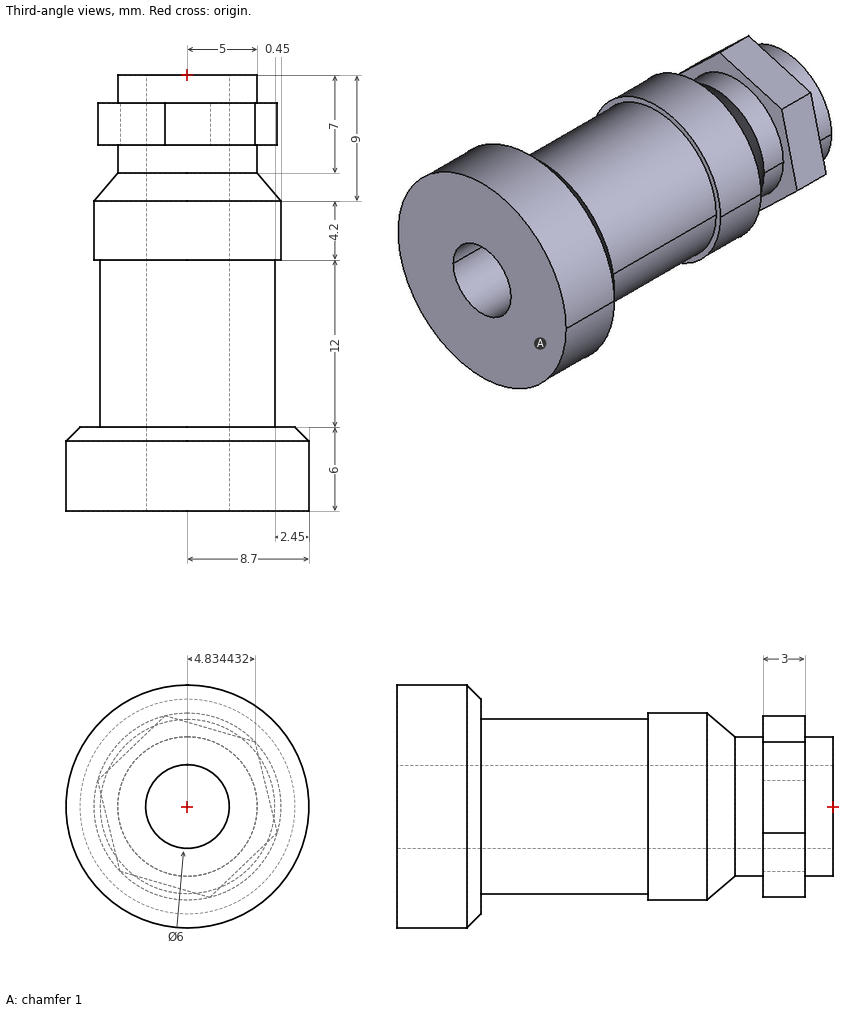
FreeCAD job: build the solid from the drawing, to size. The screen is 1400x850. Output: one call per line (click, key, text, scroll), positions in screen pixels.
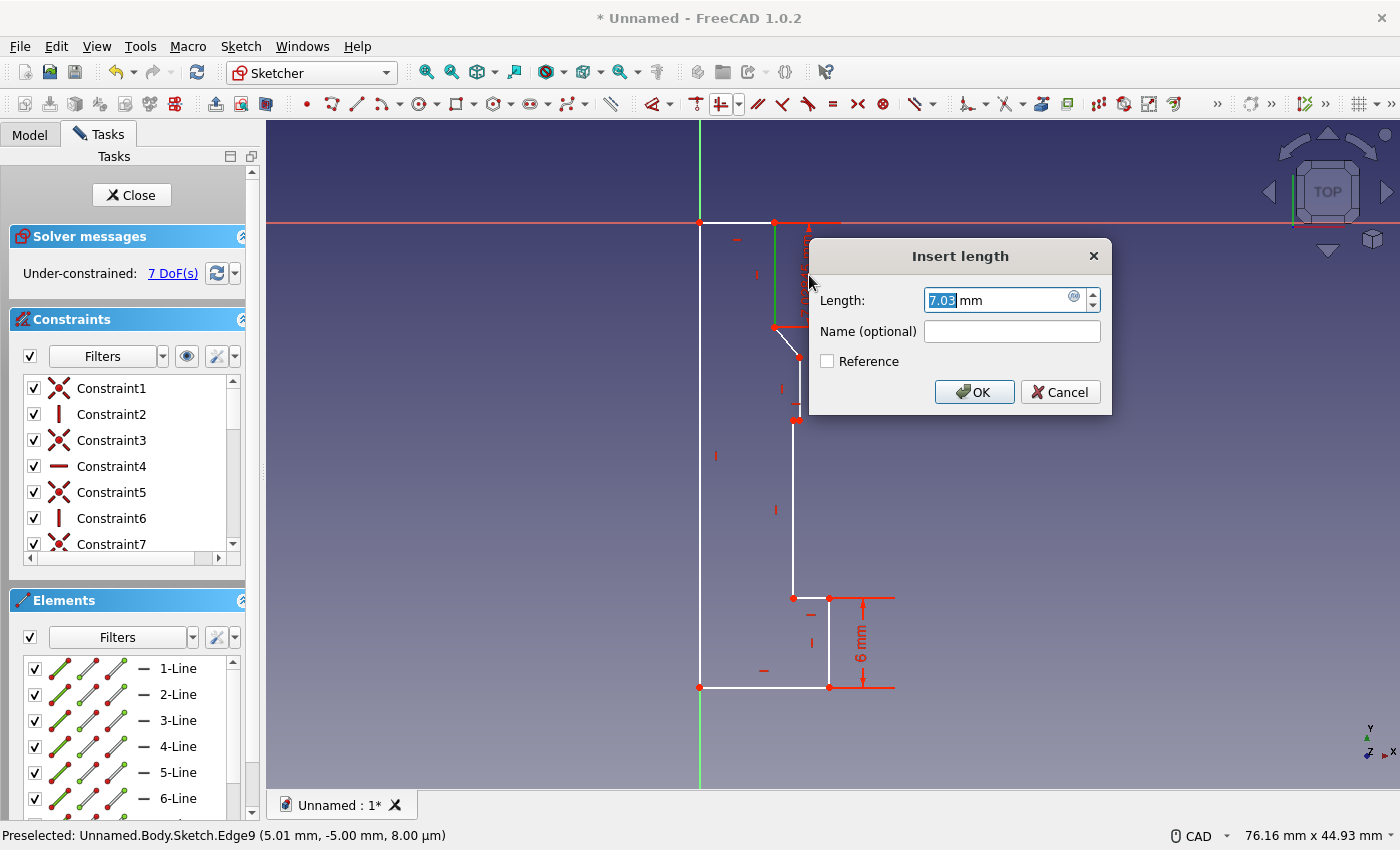
text(7)
key(Return)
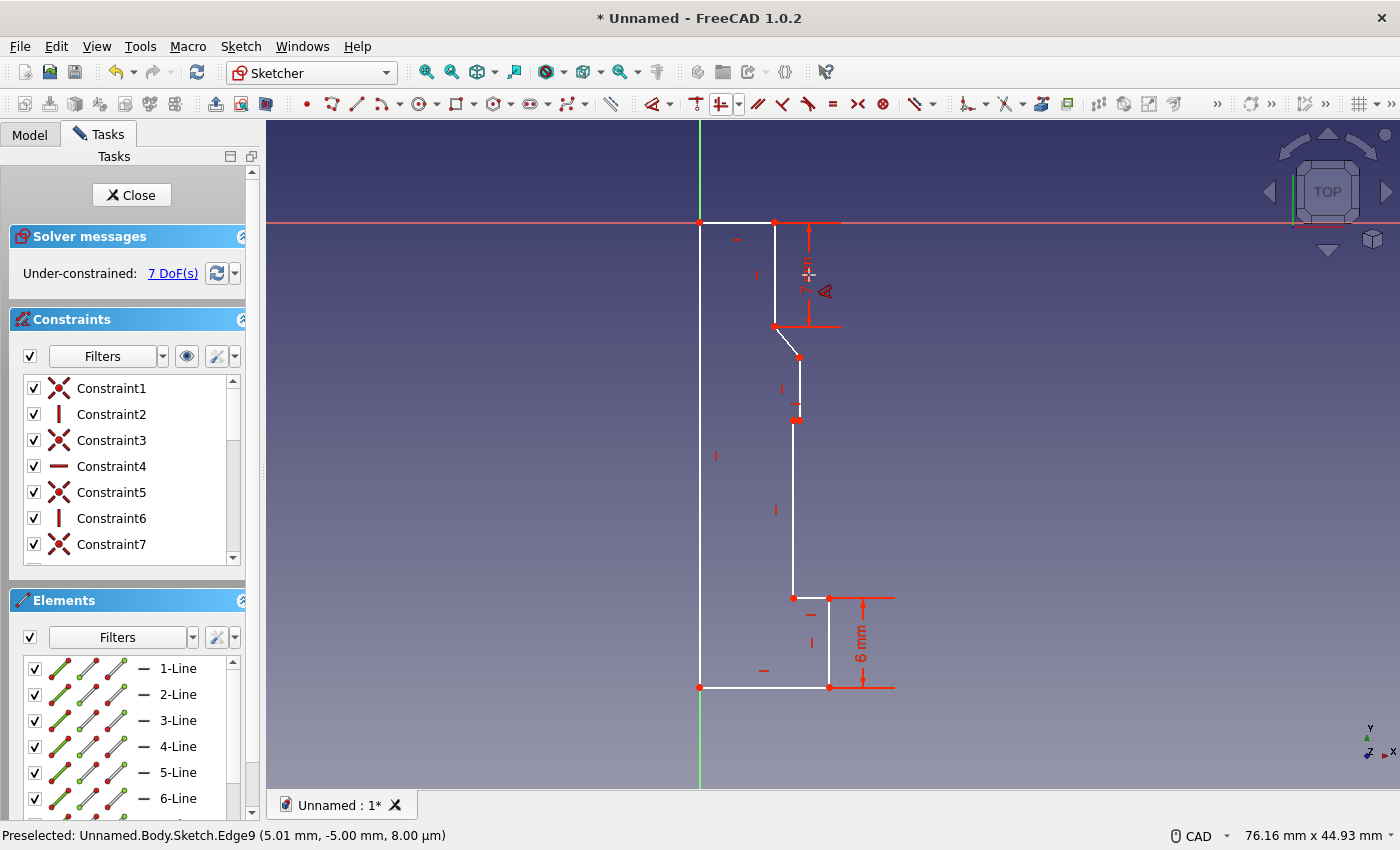
click(752, 223)
click(737, 189)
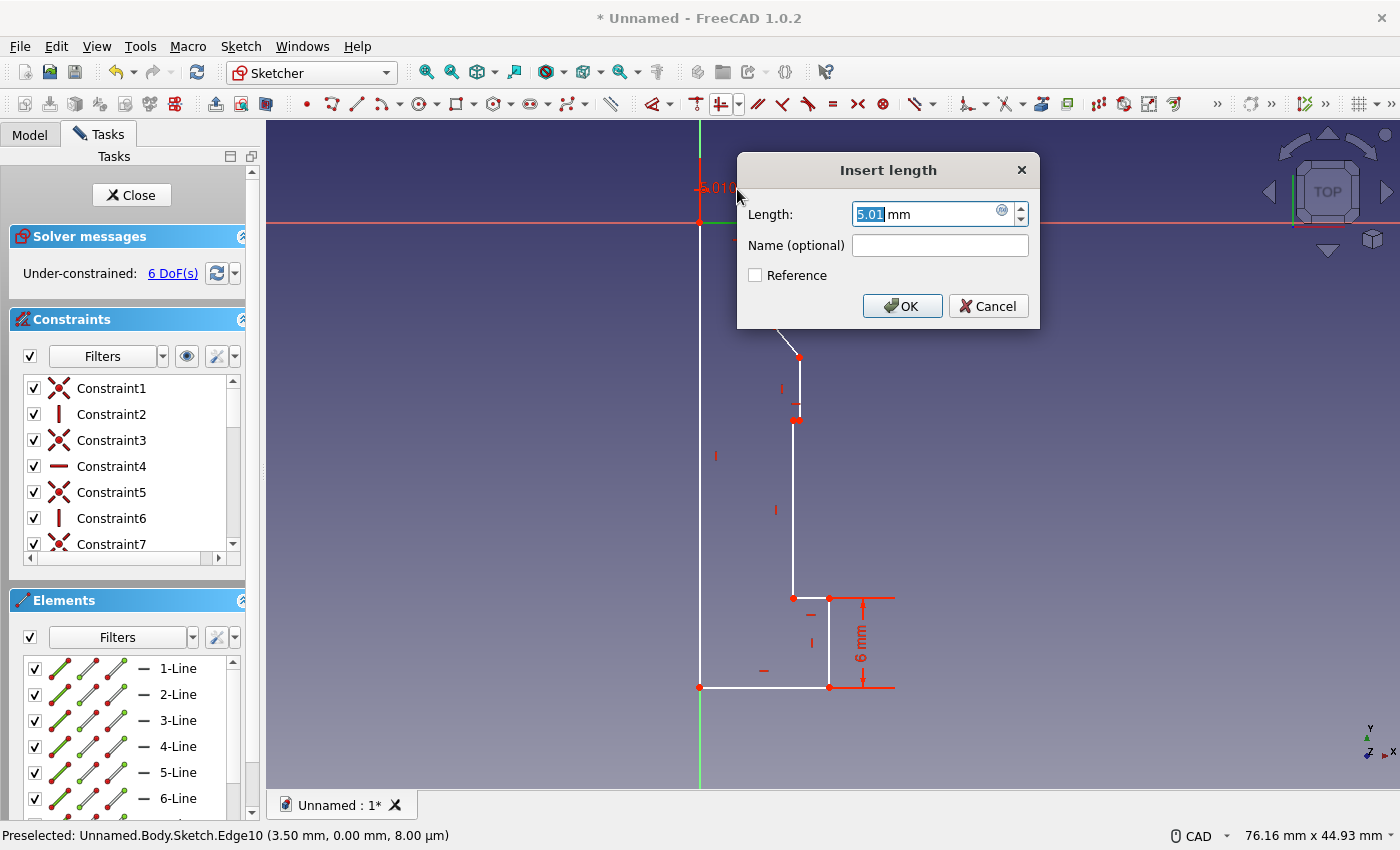
text(5)
key(Return)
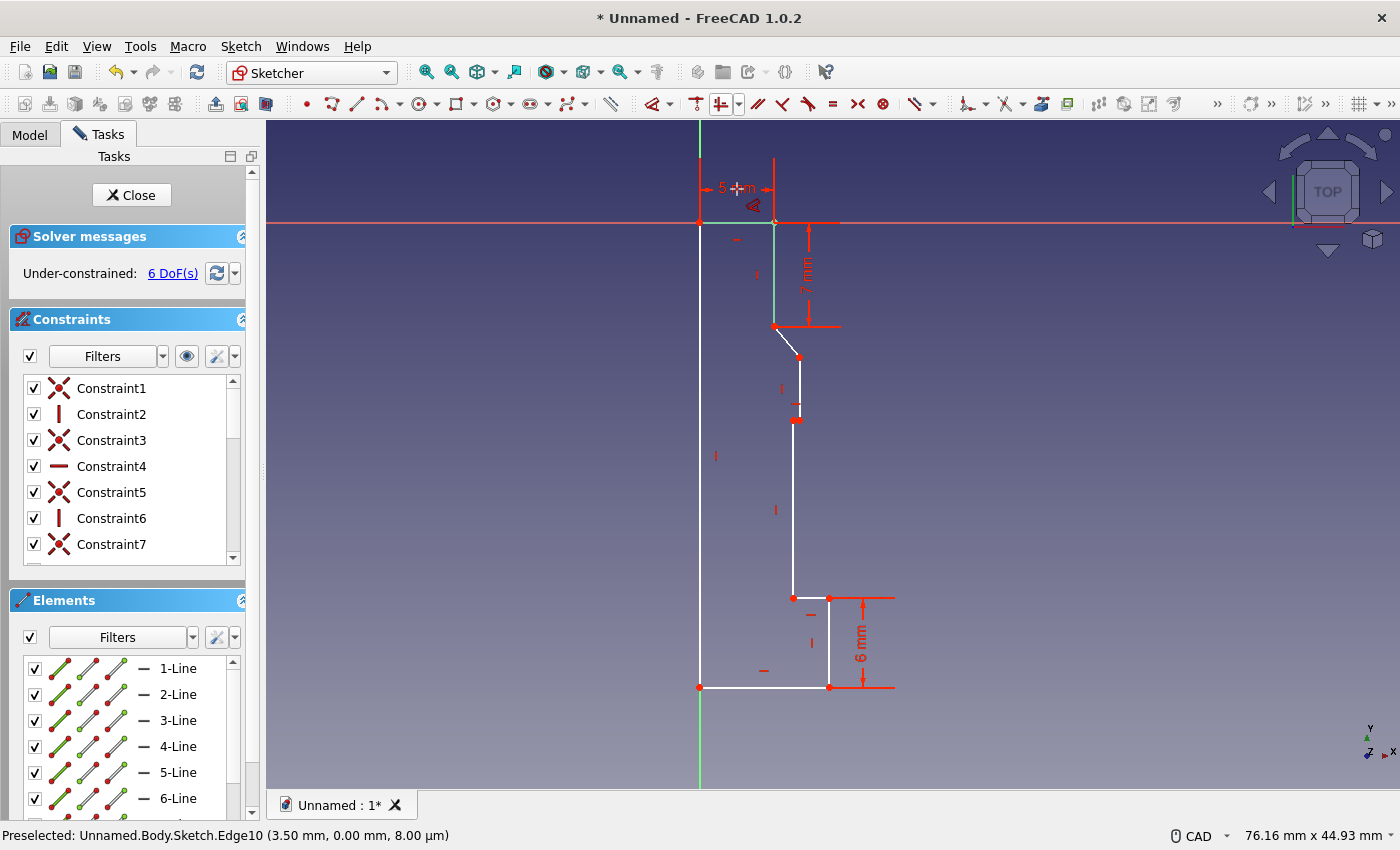
click(793, 545)
click(827, 509)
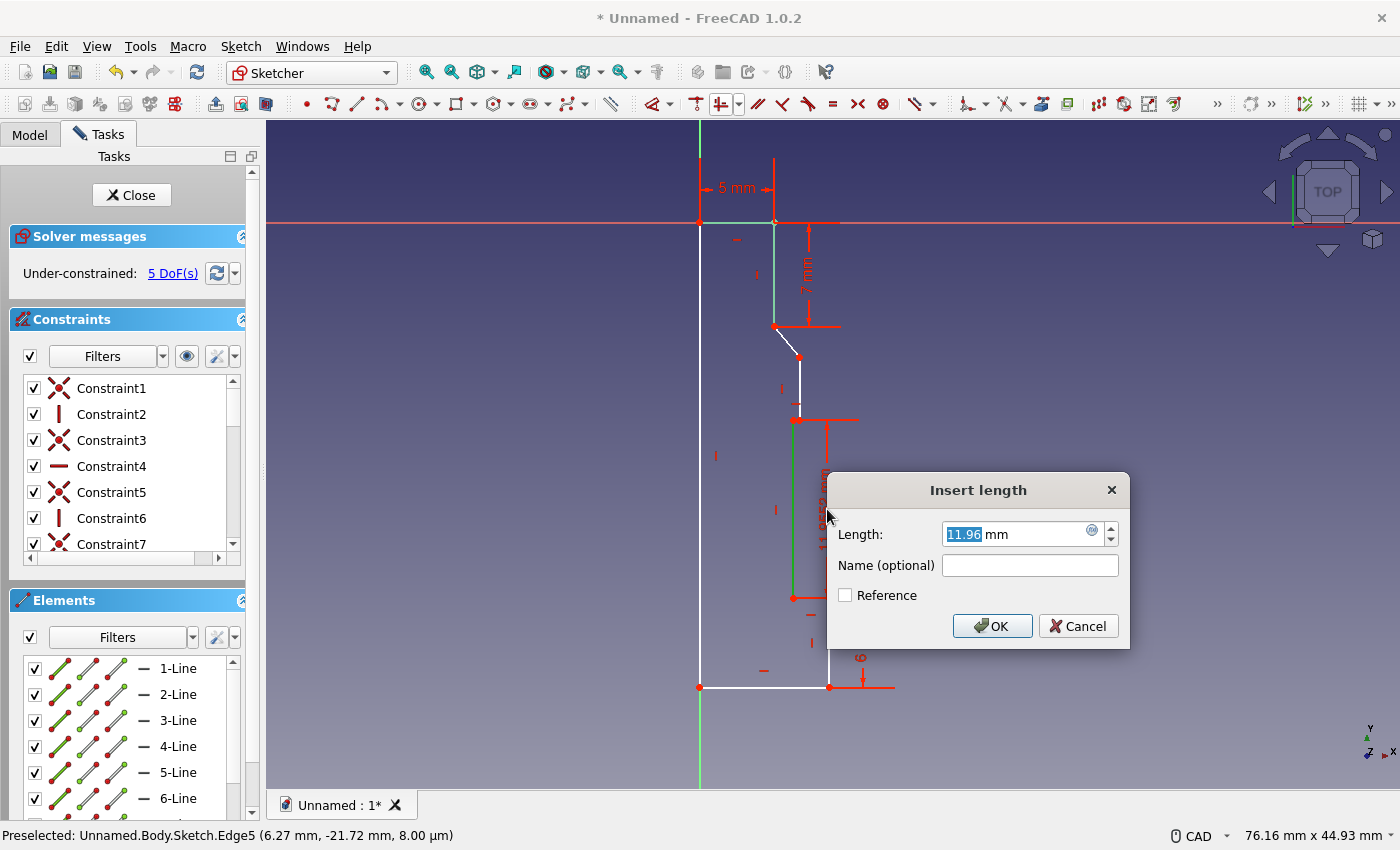
text(12)
key(Return)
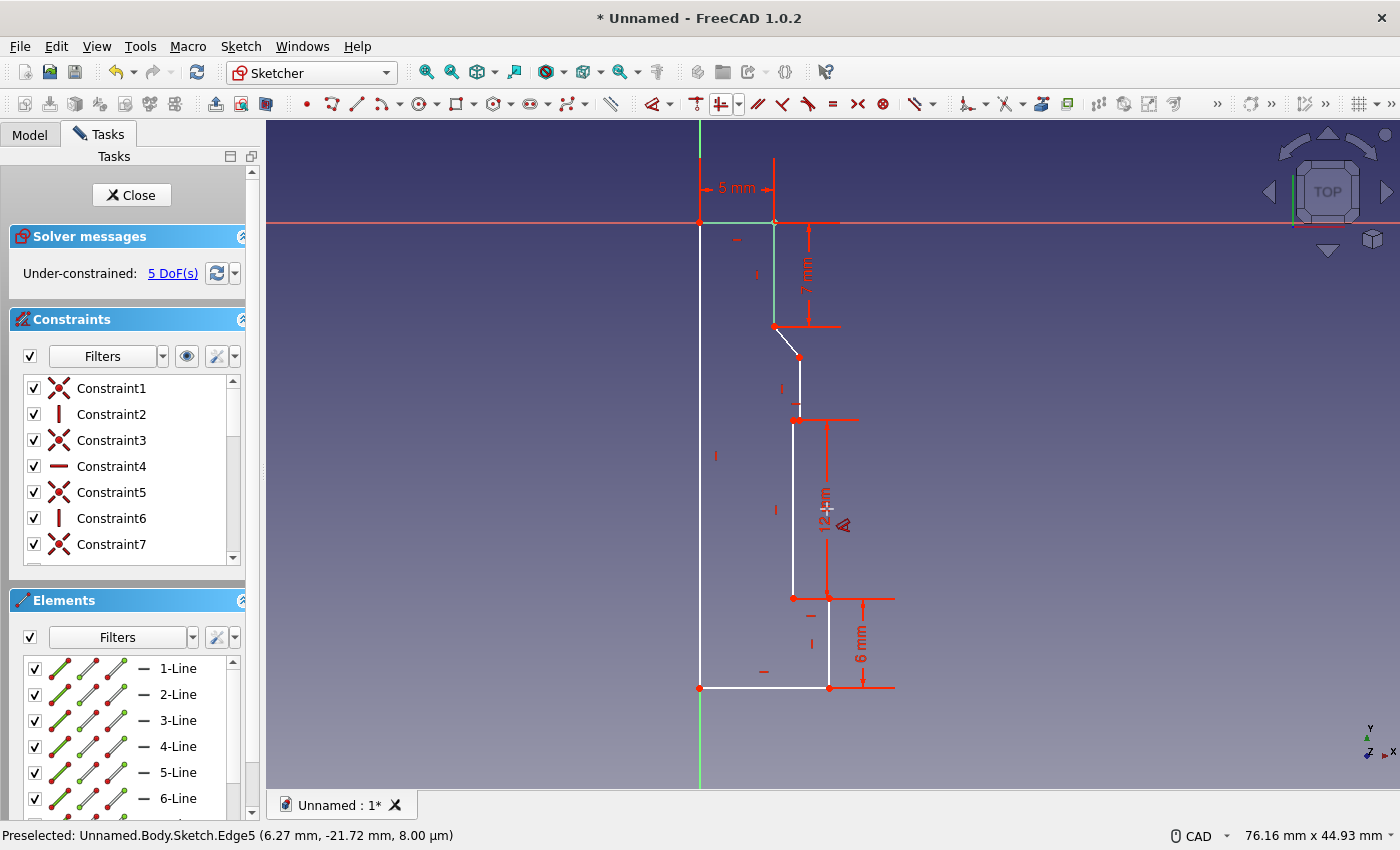
click(800, 357)
click(666, 290)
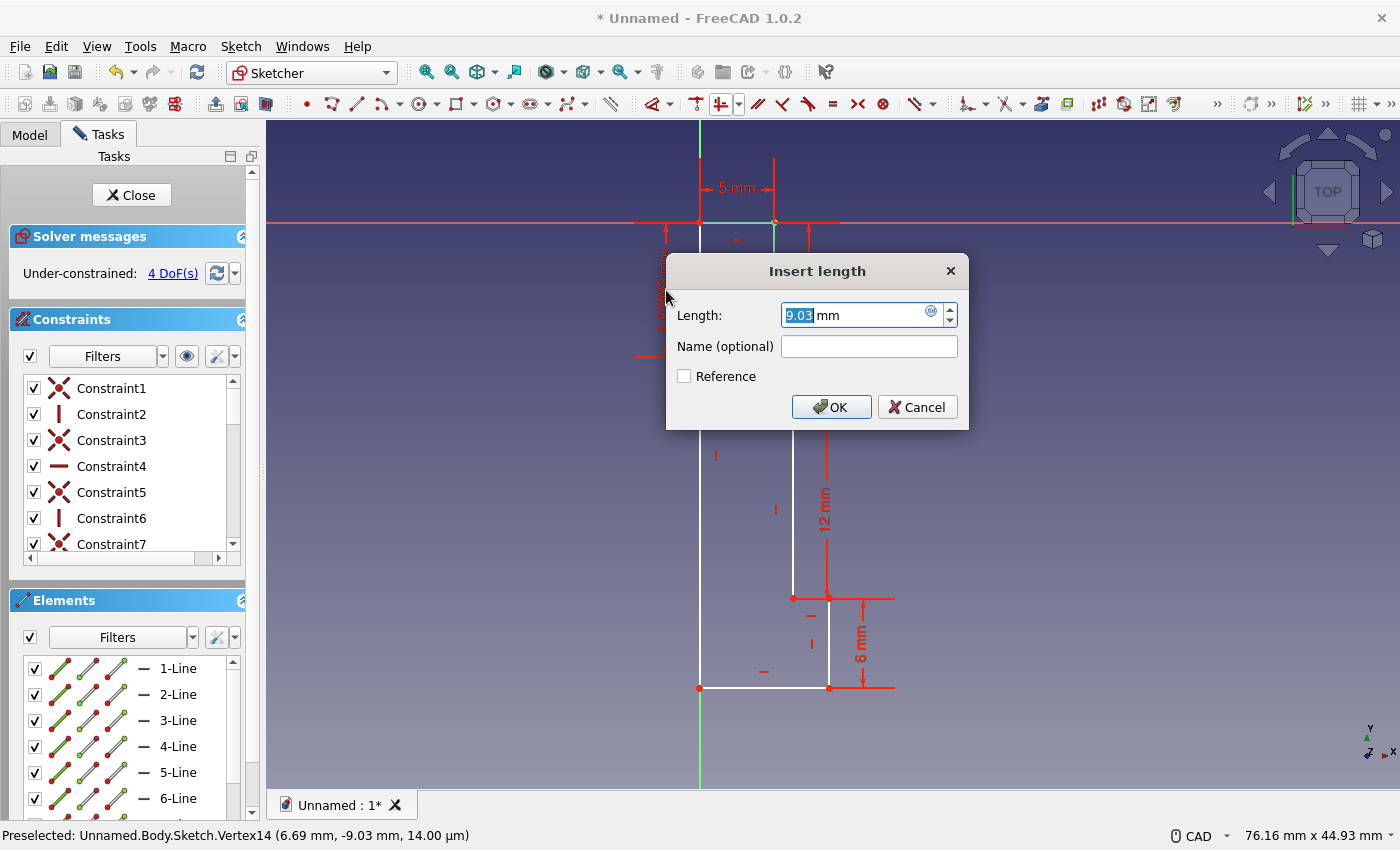
text(9)
key(Return)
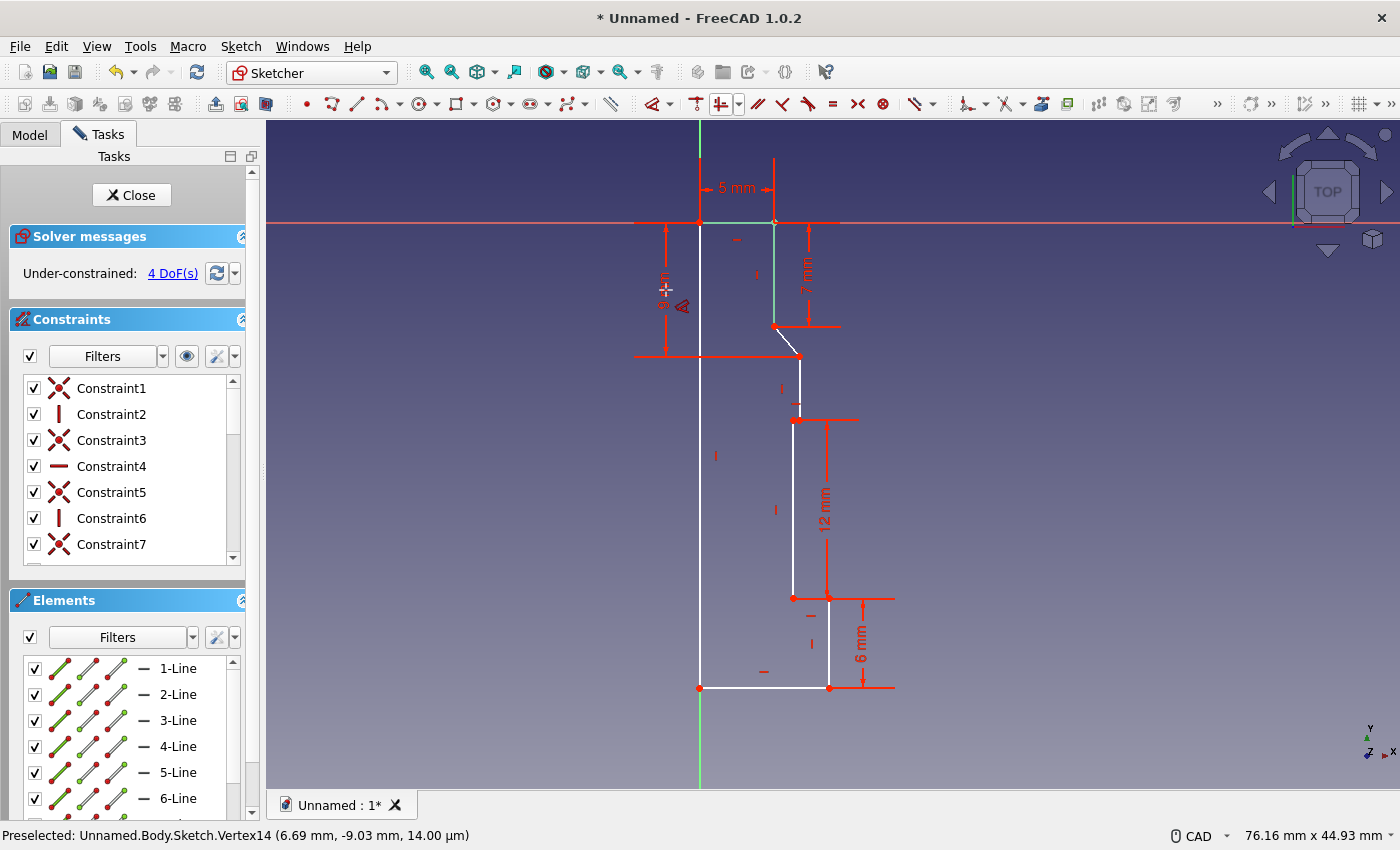
click(739, 688)
click(765, 722)